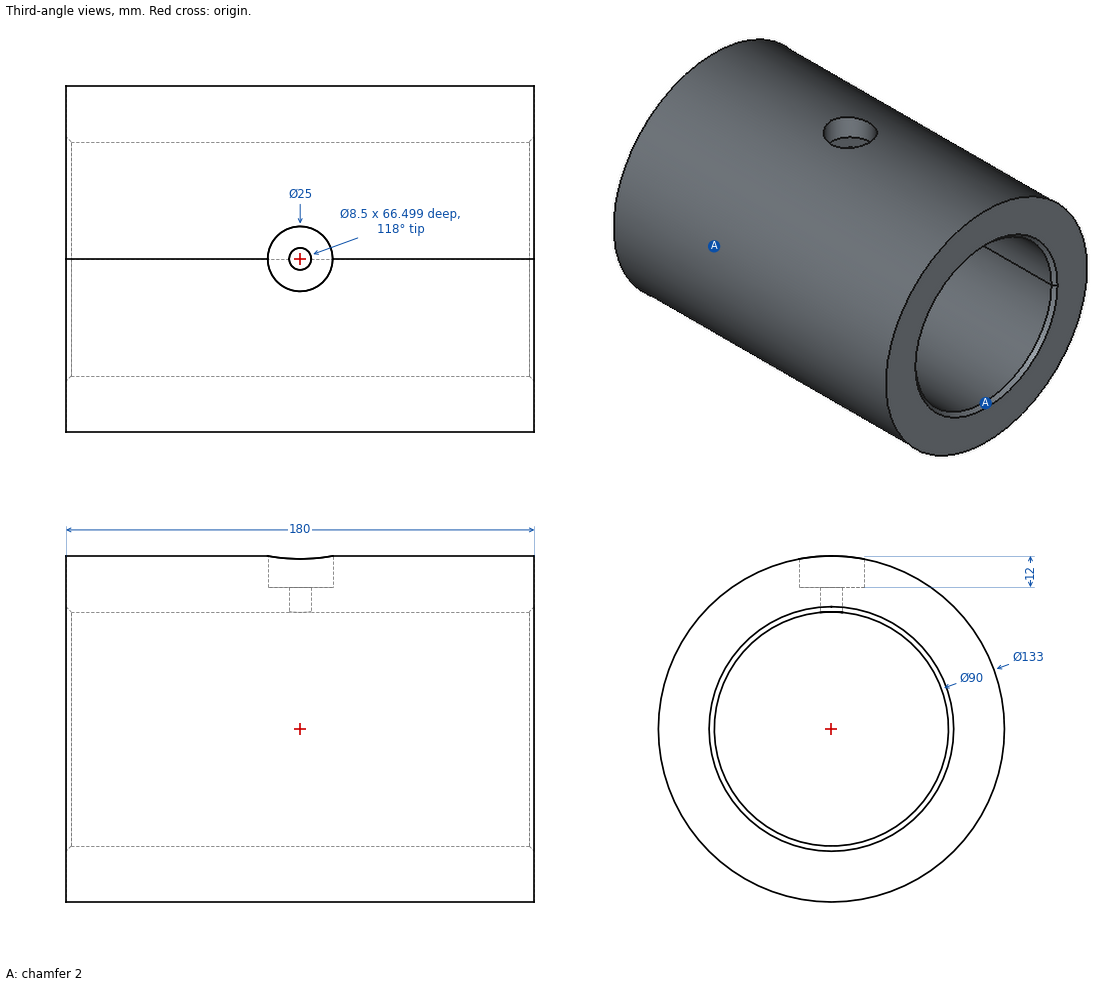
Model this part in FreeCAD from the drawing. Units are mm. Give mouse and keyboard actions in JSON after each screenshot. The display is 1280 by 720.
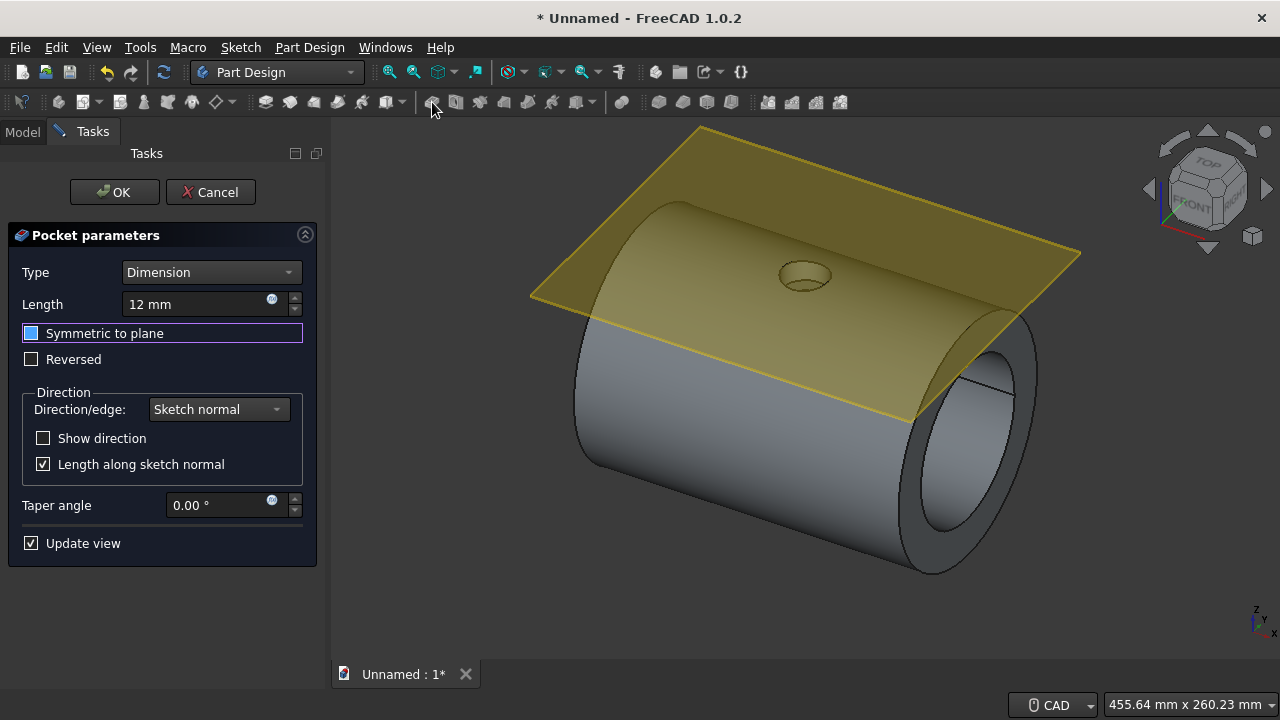
{"action": "left_click", "coordinate": [115, 192]}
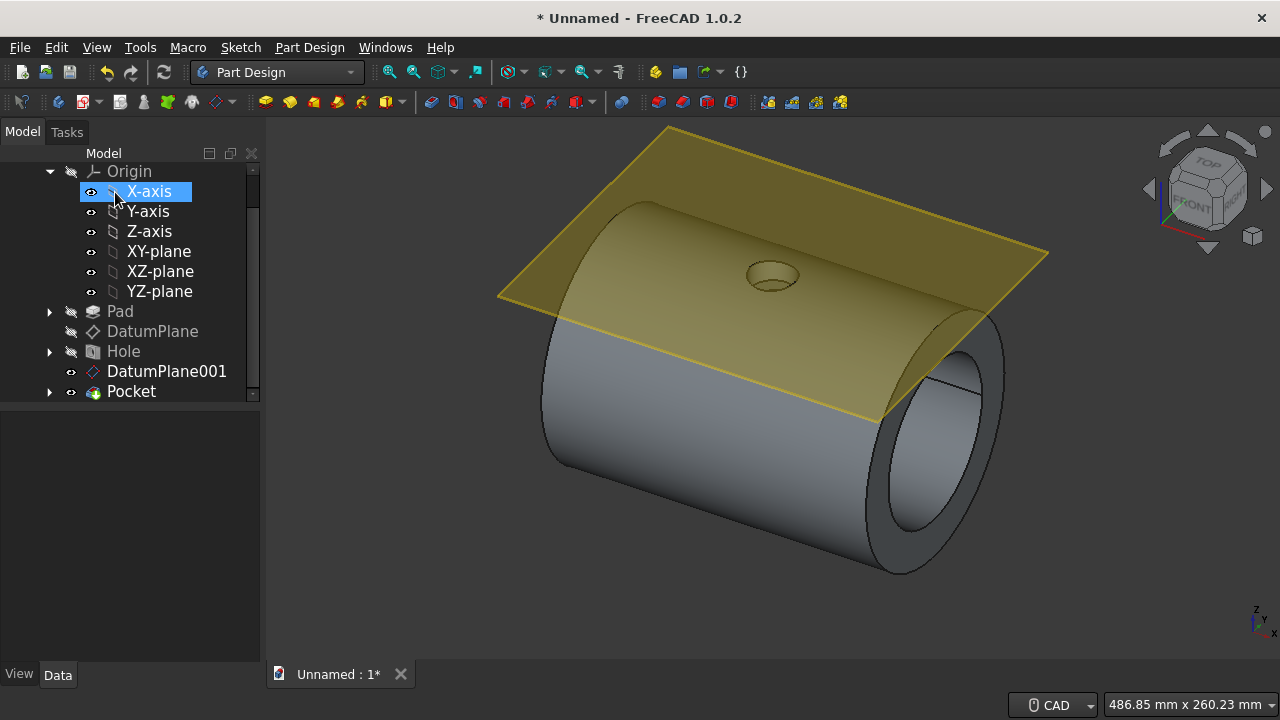
{"action": "left_click", "coordinate": [116, 372]}
{"action": "key", "text": "space"}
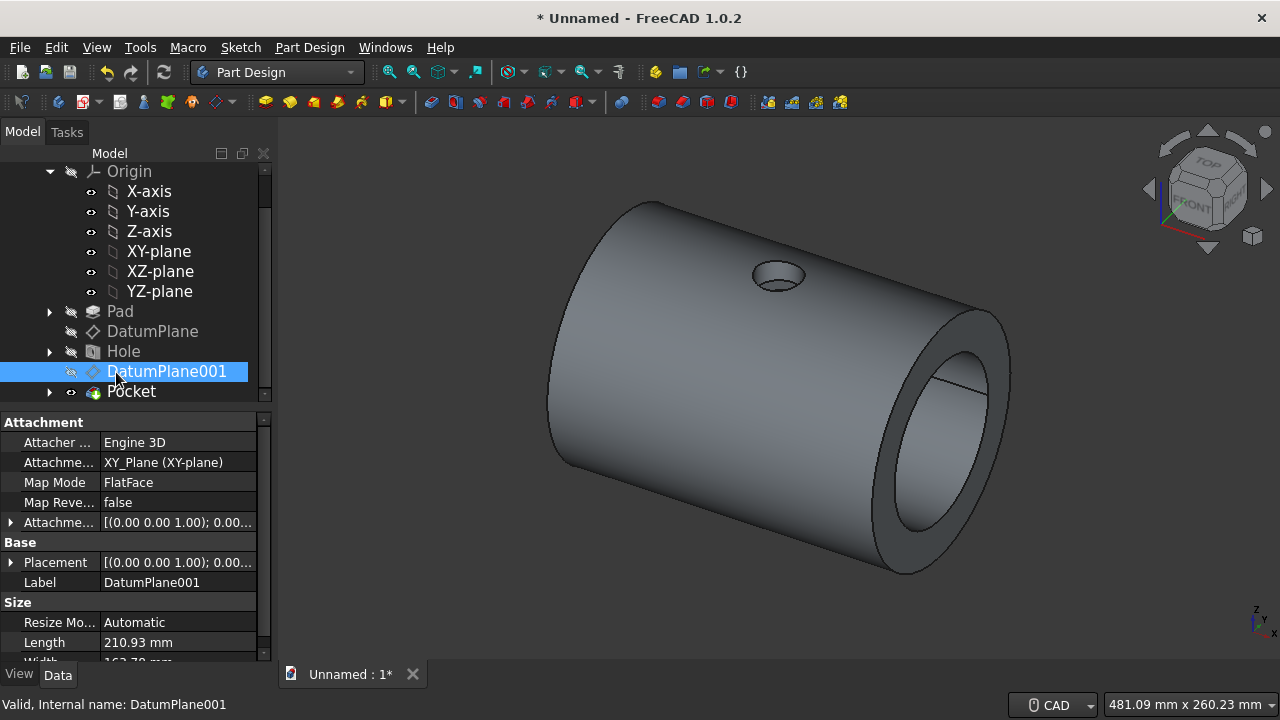
{"action": "left_click", "coordinate": [927, 528]}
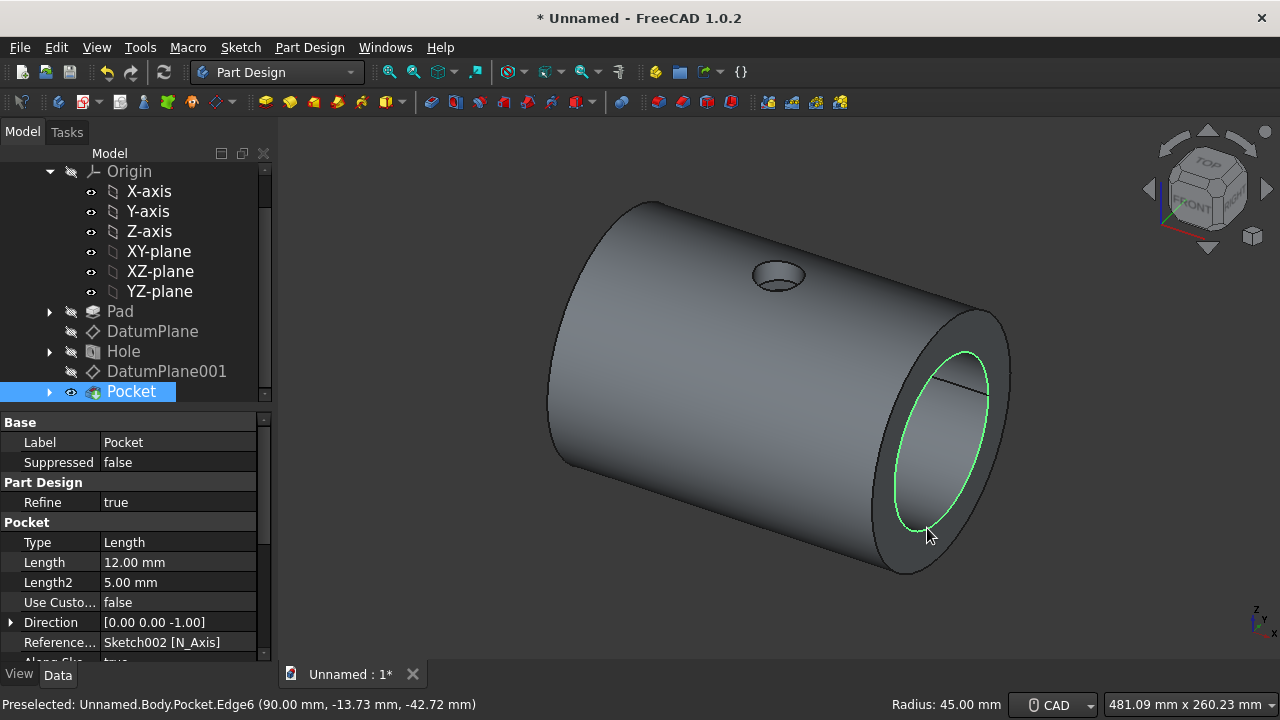
{"action": "key", "text": "0"}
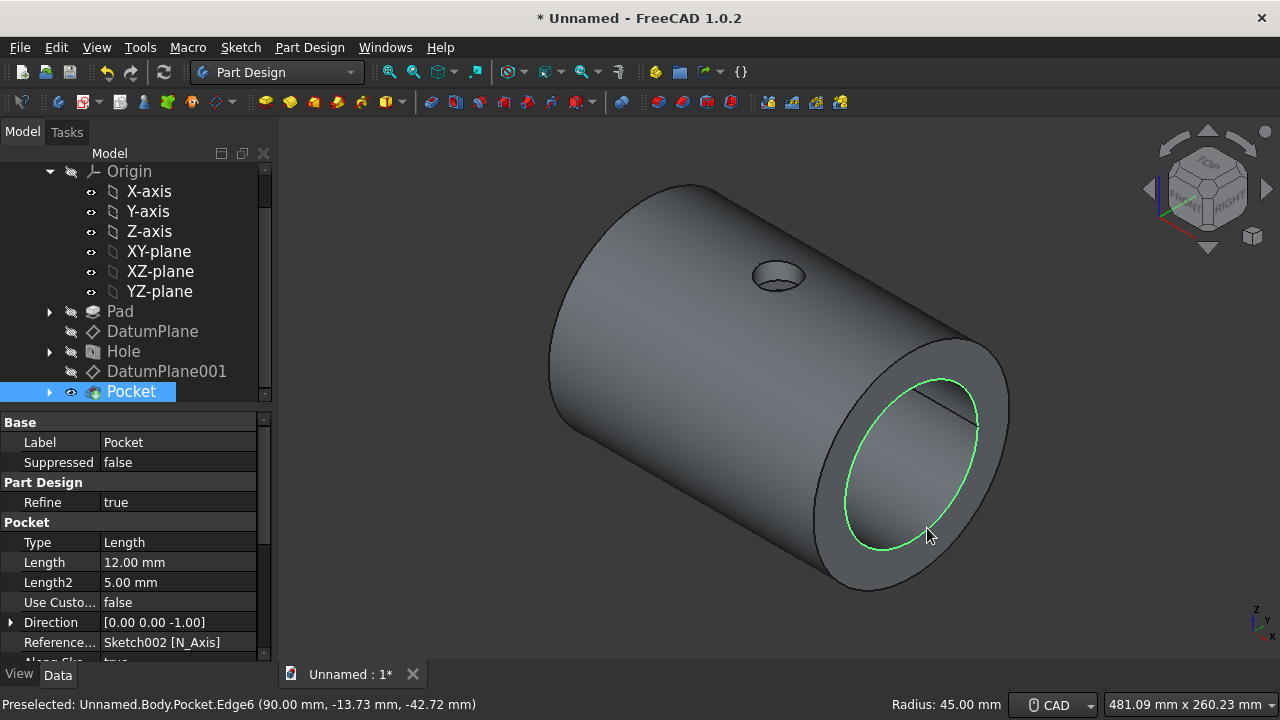
{"action": "key", "text": "2"}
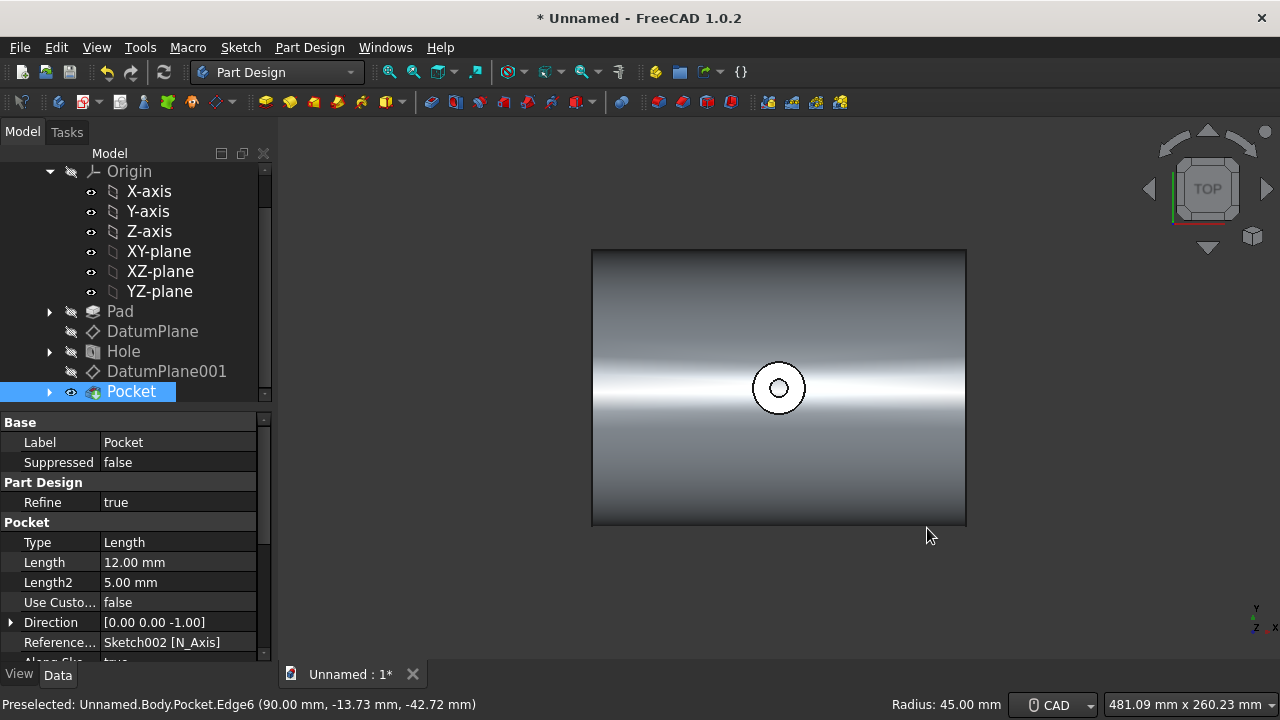
{"action": "key", "text": "1"}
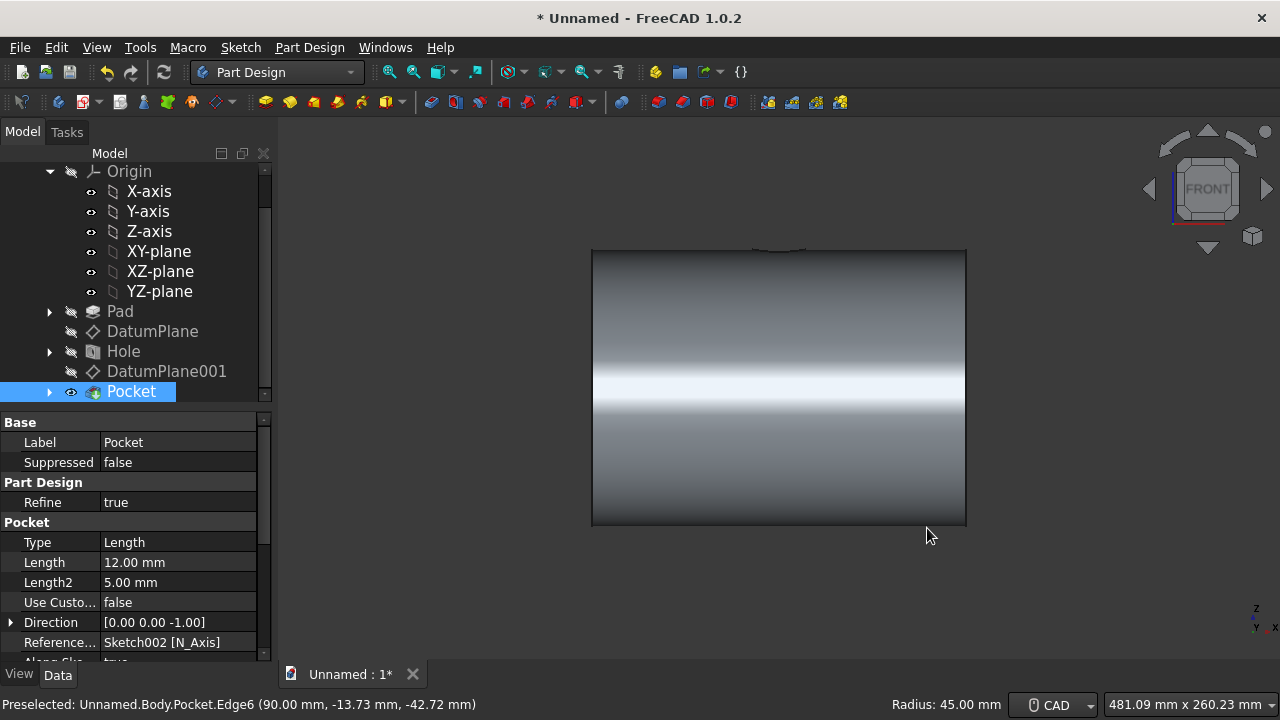
{"action": "key", "text": "3"}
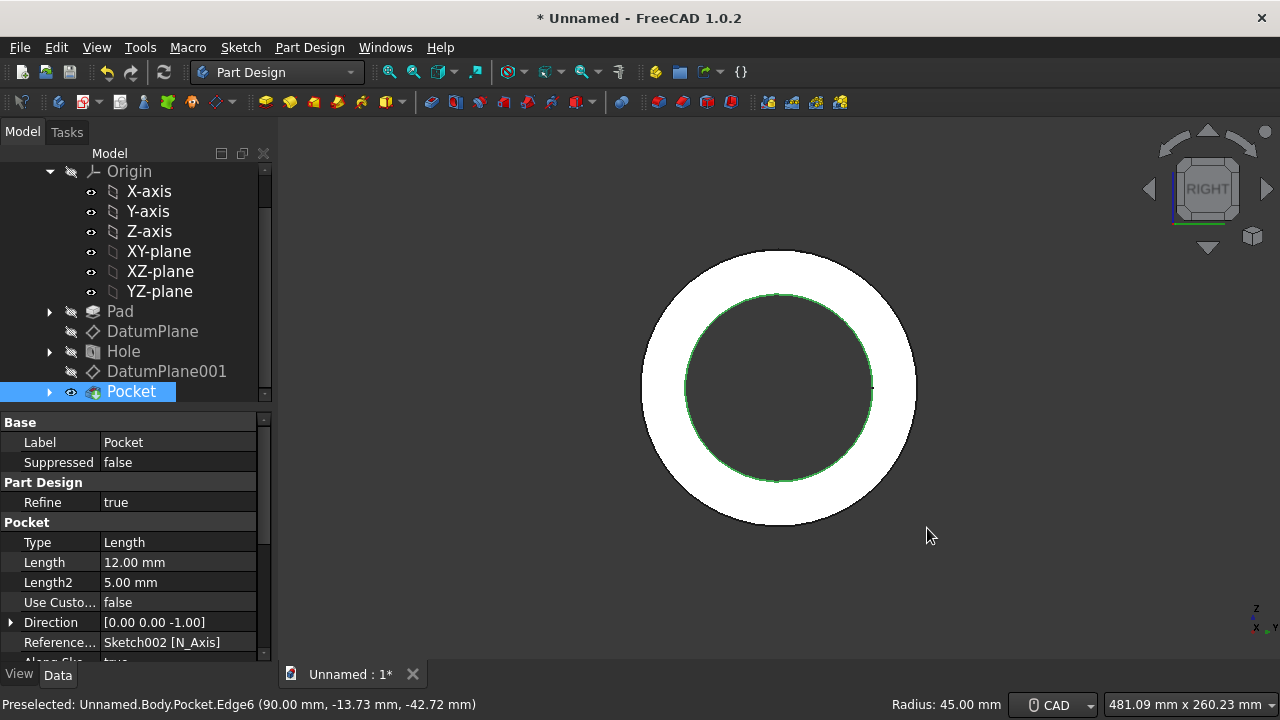
{"action": "key", "text": "5"}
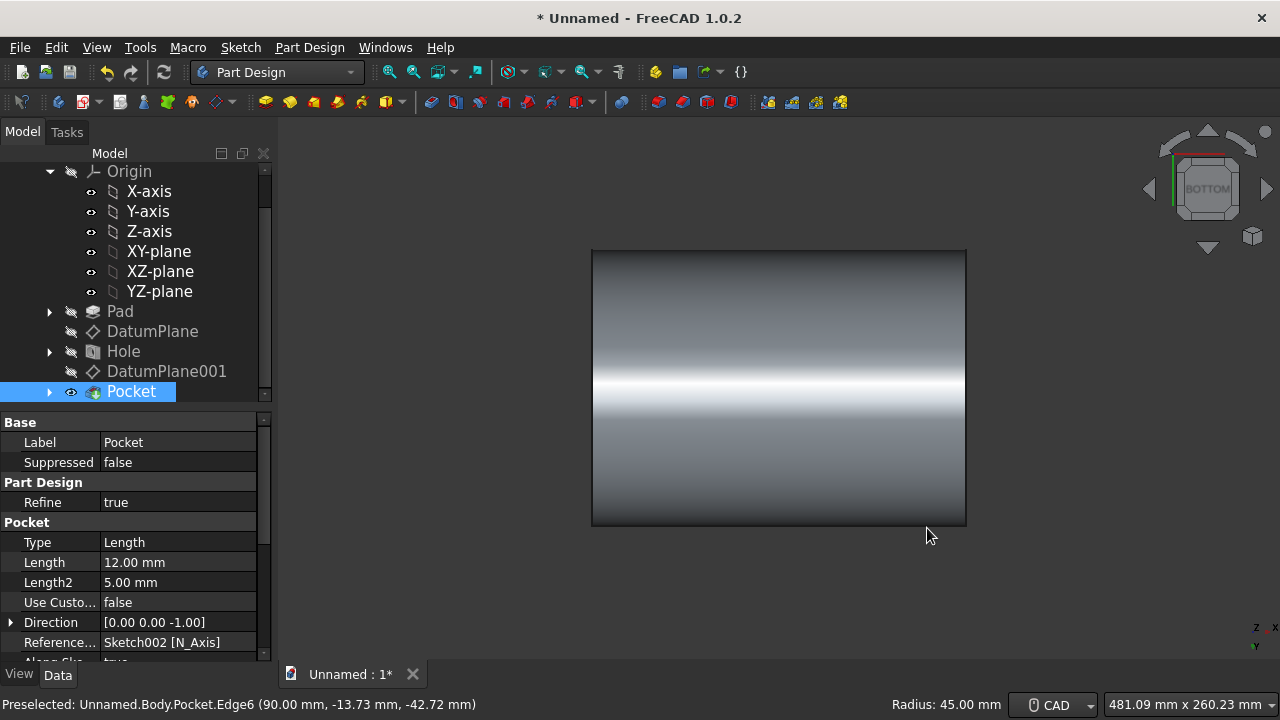
{"action": "key", "text": "4"}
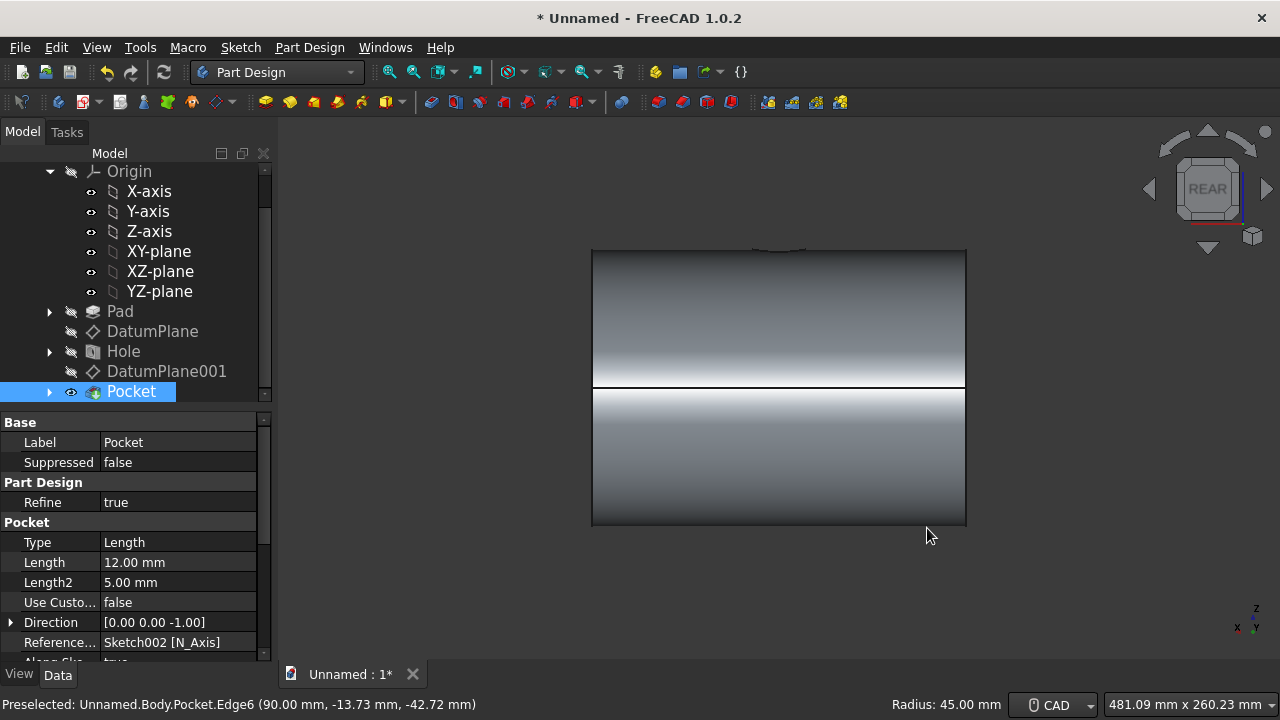
{"action": "key", "text": "6"}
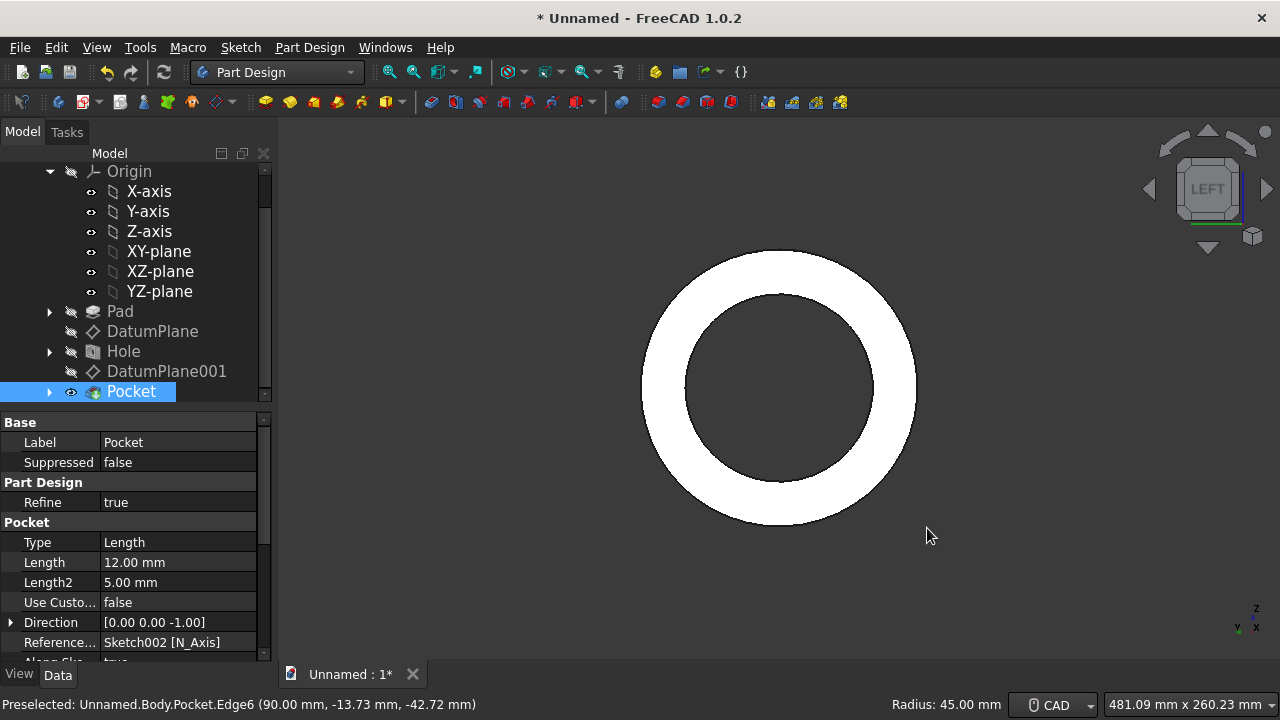
{"action": "left_click", "coordinate": [873, 387], "text": "ctrl"}